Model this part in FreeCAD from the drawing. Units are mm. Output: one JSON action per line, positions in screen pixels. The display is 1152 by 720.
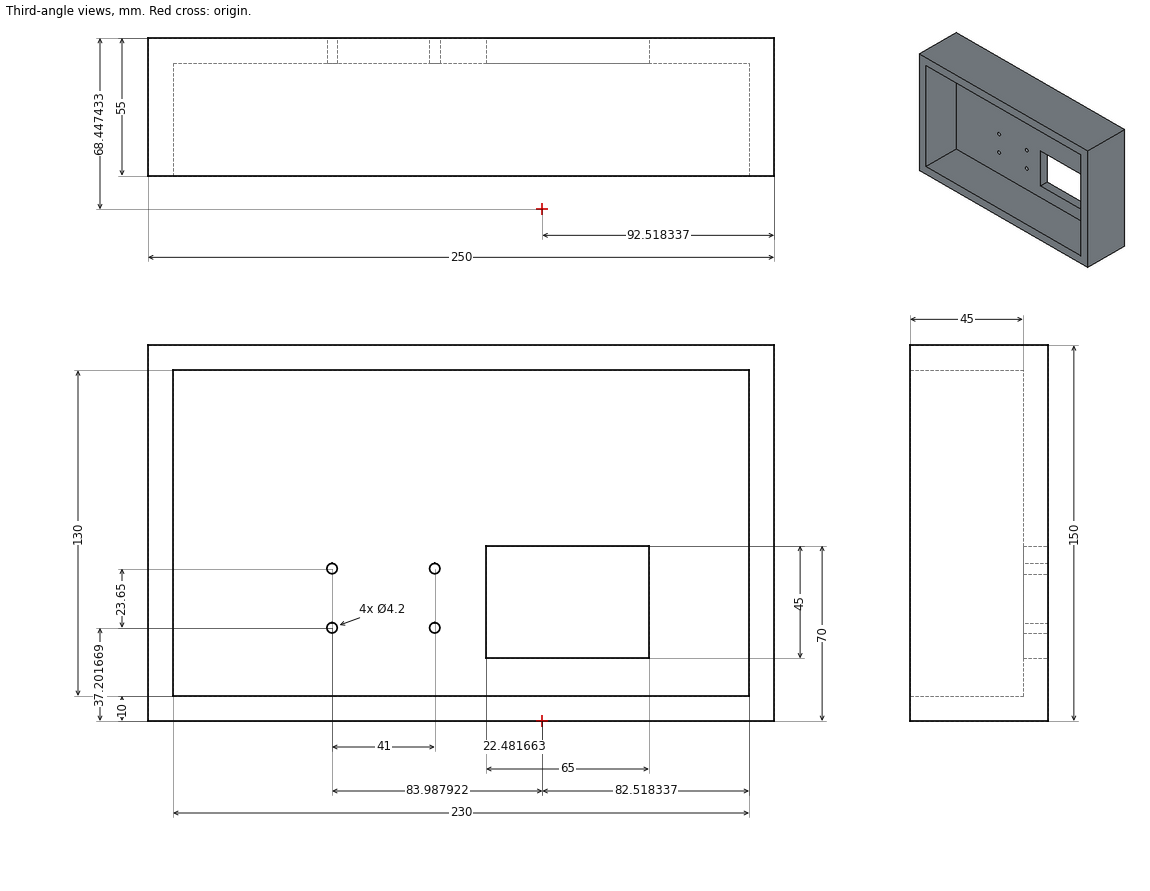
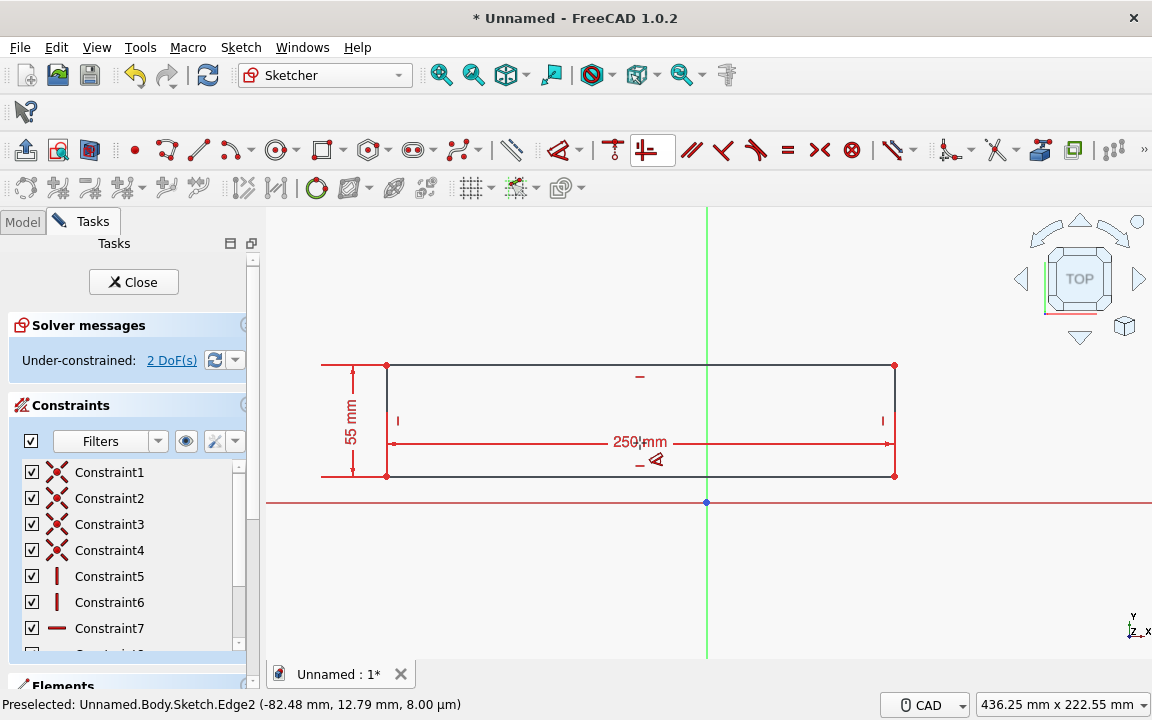
{"action": "left_click", "coordinate": [387, 365]}
{"action": "left_click", "coordinate": [353, 466]}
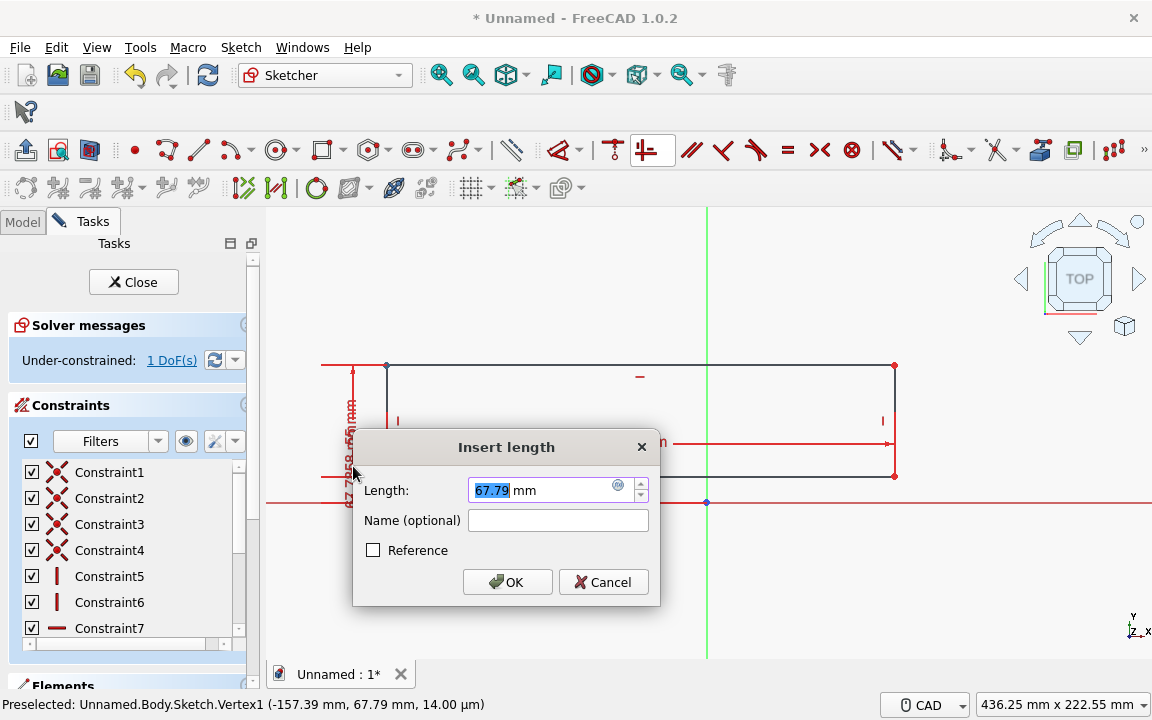
{"action": "type", "text": "68.447433"}
{"action": "key", "text": "Return"}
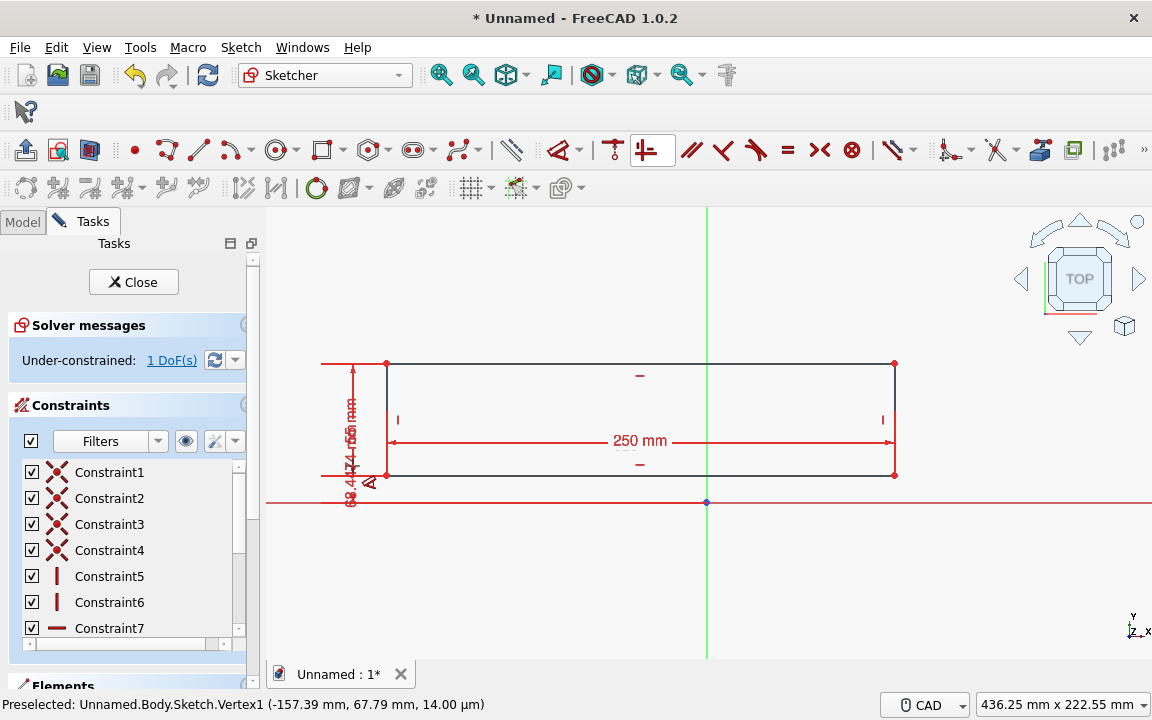
{"action": "left_click", "coordinate": [895, 476]}
{"action": "left_click", "coordinate": [801, 537]}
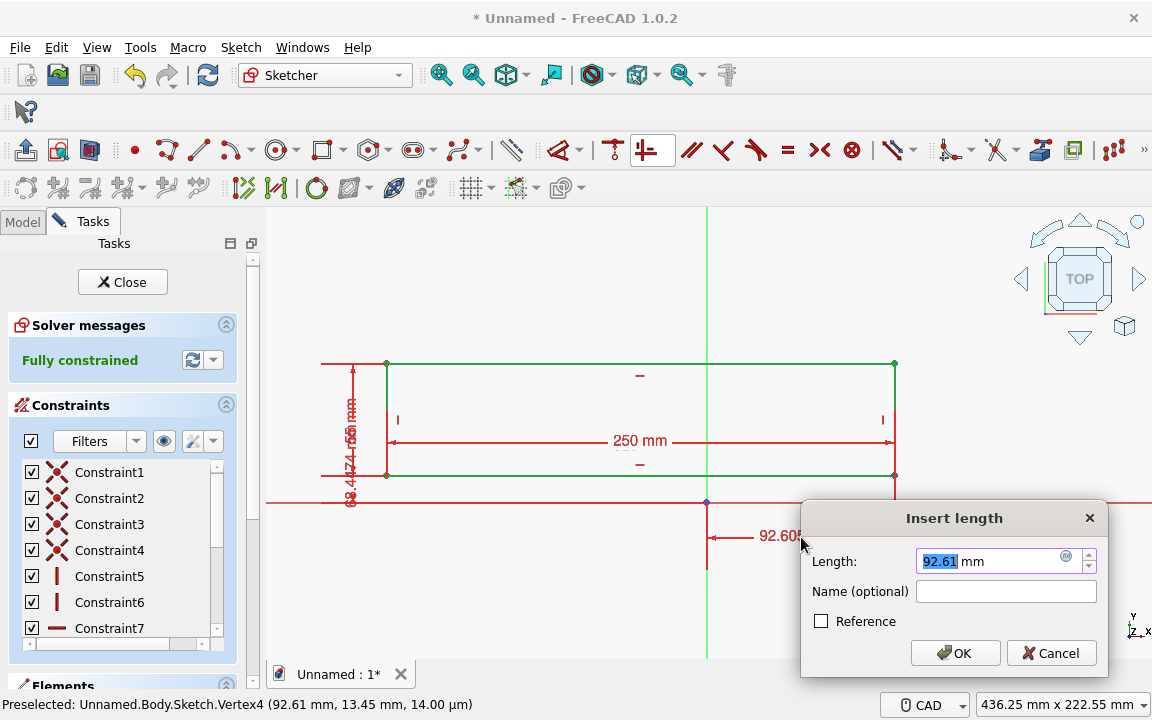
{"action": "type", "text": "92.518337"}
{"action": "key", "text": "Return"}
{"action": "key", "text": "Escape"}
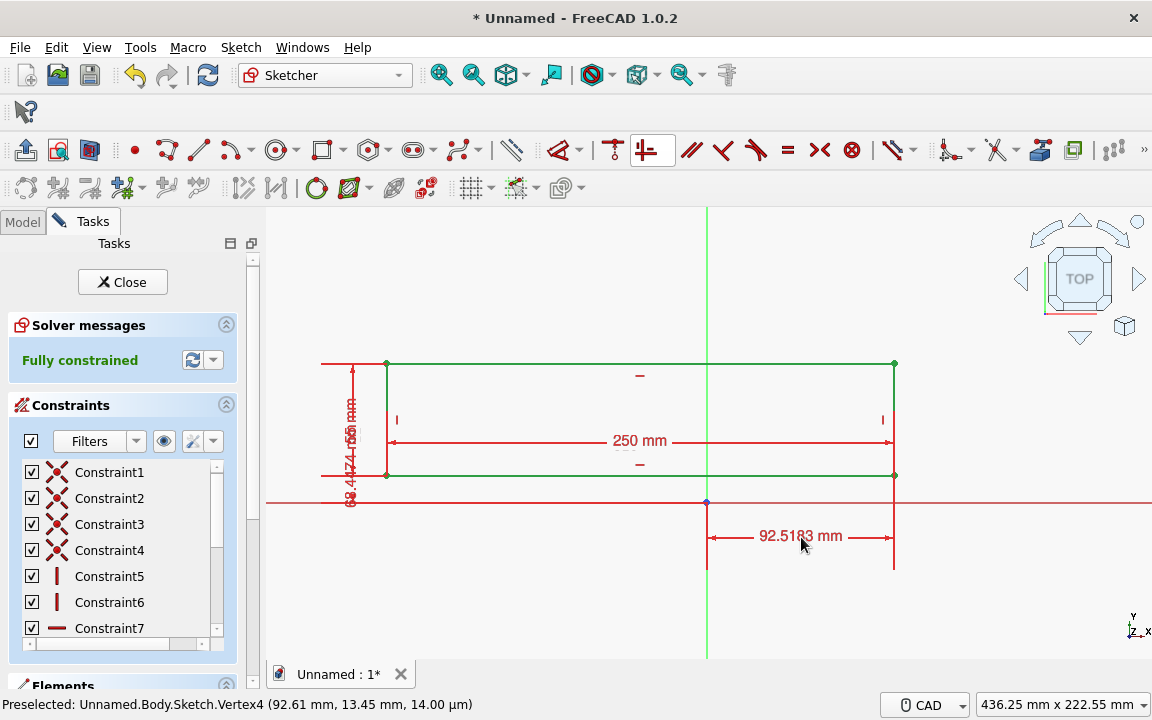
{"action": "left_click", "coordinate": [123, 282]}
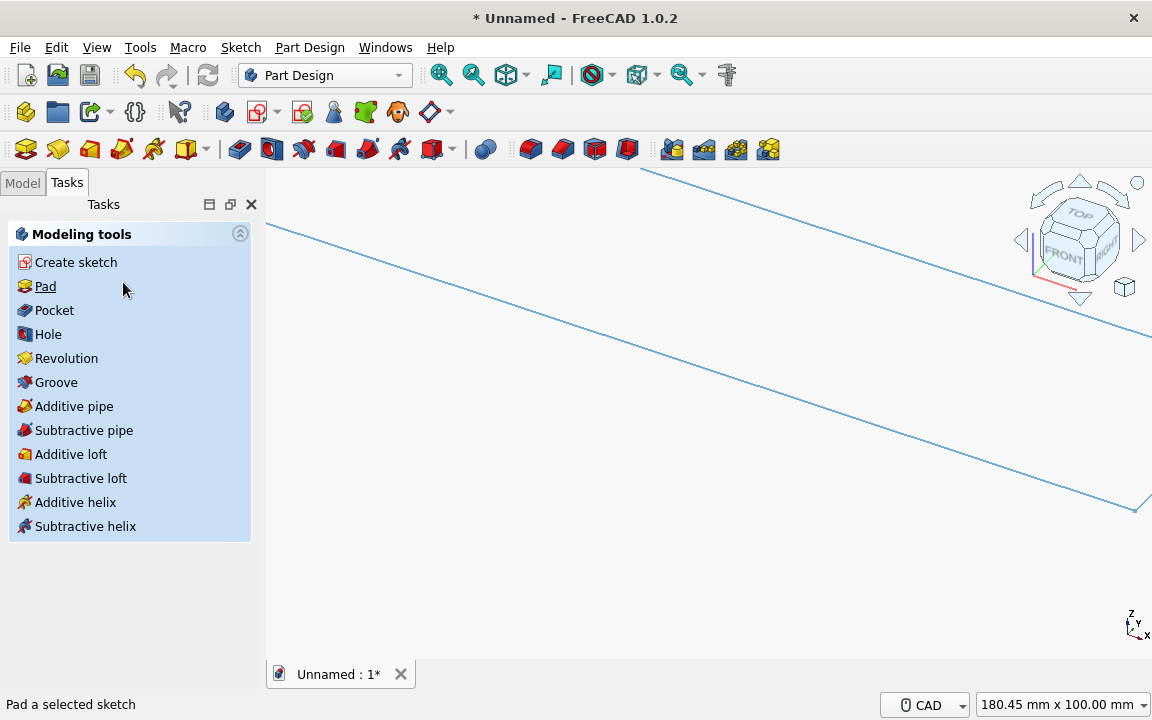
{"action": "left_click", "coordinate": [26, 150]}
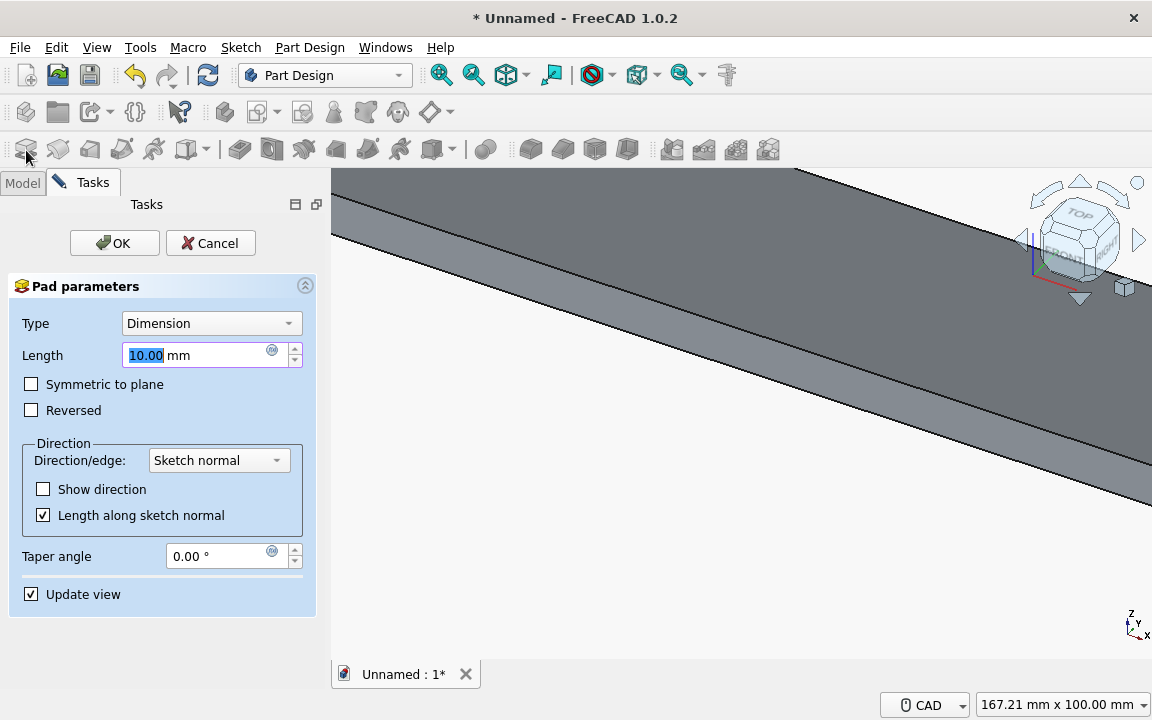
{"action": "type", "text": "150"}
{"action": "key", "text": "Tab"}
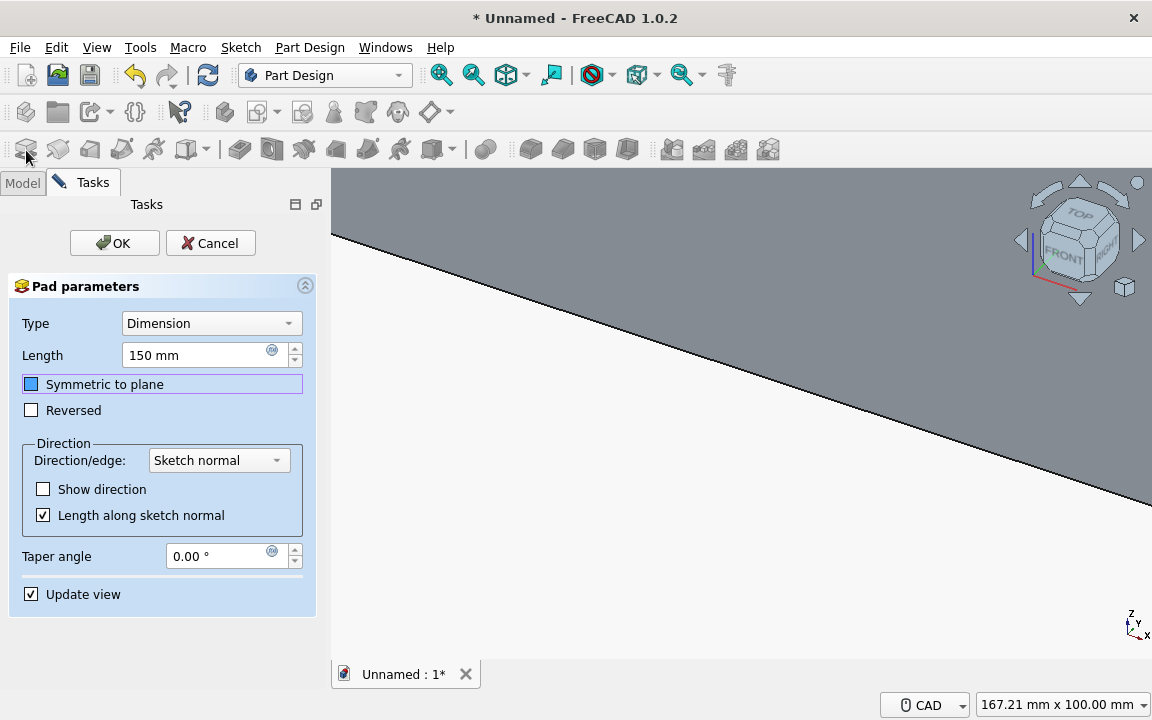
{"action": "left_click", "coordinate": [115, 243]}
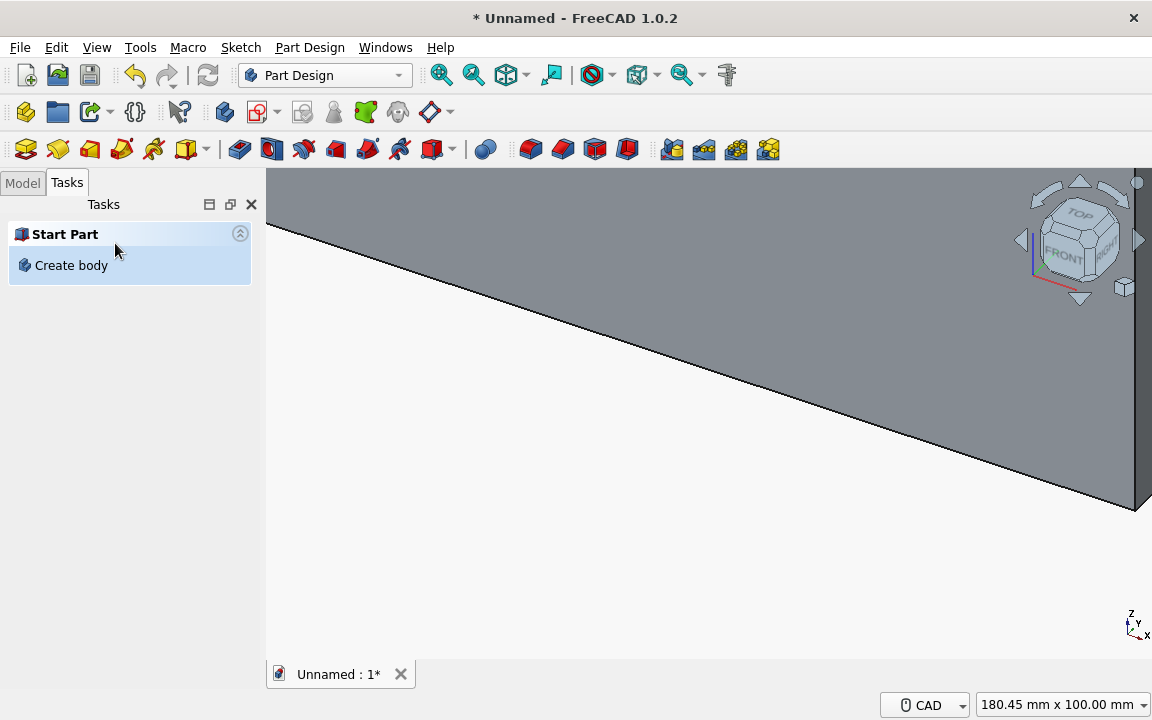
{"action": "left_click", "coordinate": [442, 76]}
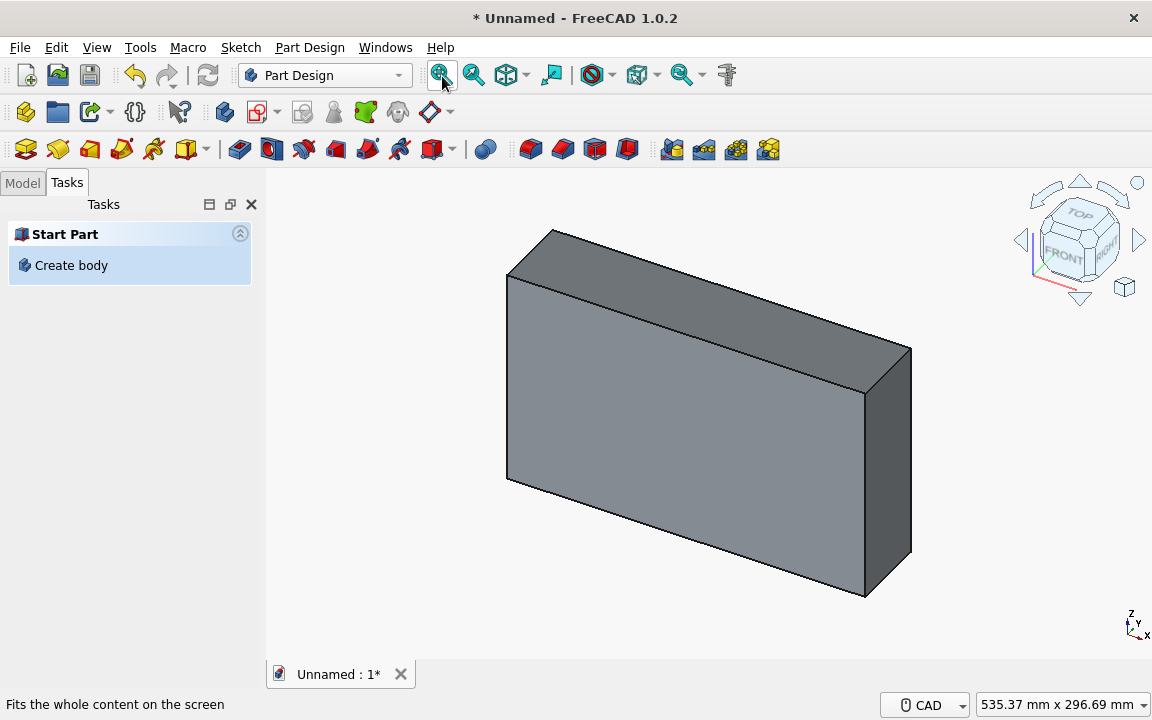
{"action": "left_click", "coordinate": [737, 452]}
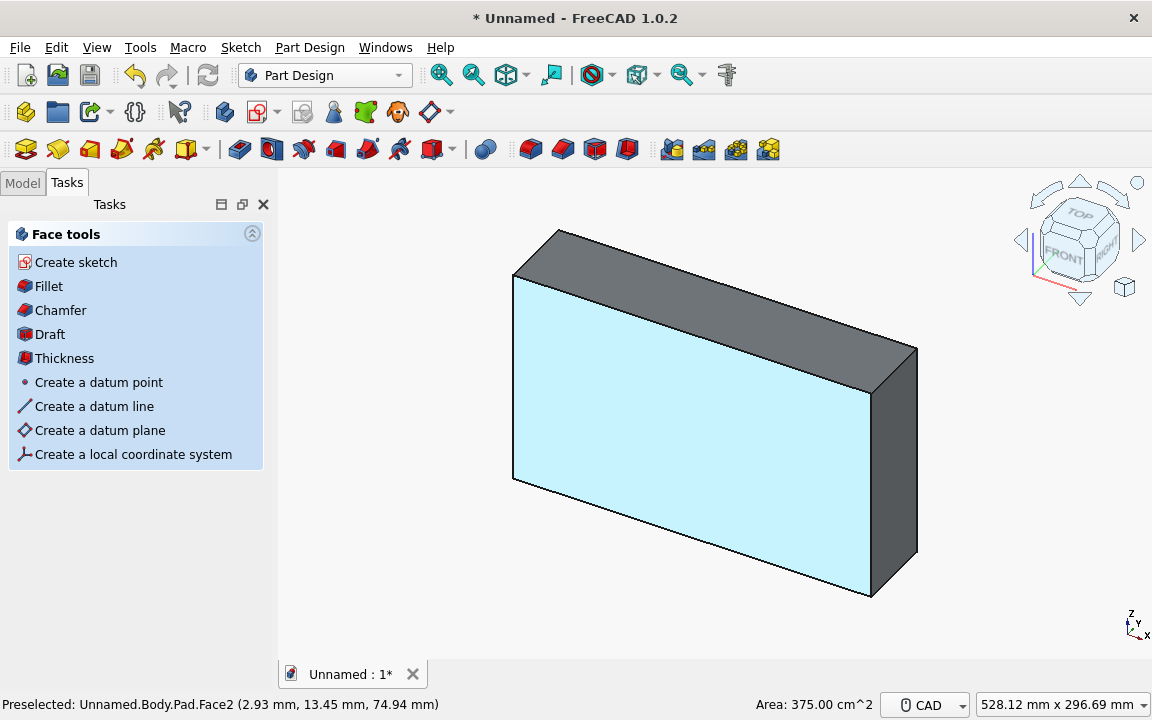
{"action": "left_click", "coordinate": [258, 112]}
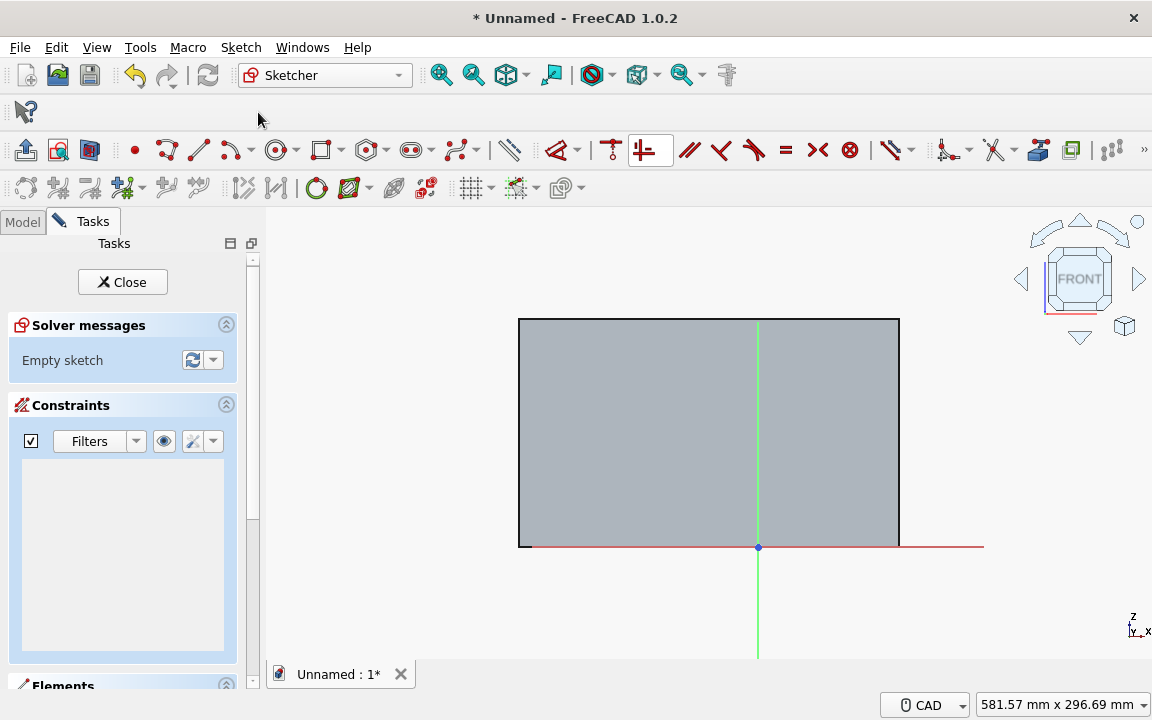
{"action": "left_click", "coordinate": [322, 150]}